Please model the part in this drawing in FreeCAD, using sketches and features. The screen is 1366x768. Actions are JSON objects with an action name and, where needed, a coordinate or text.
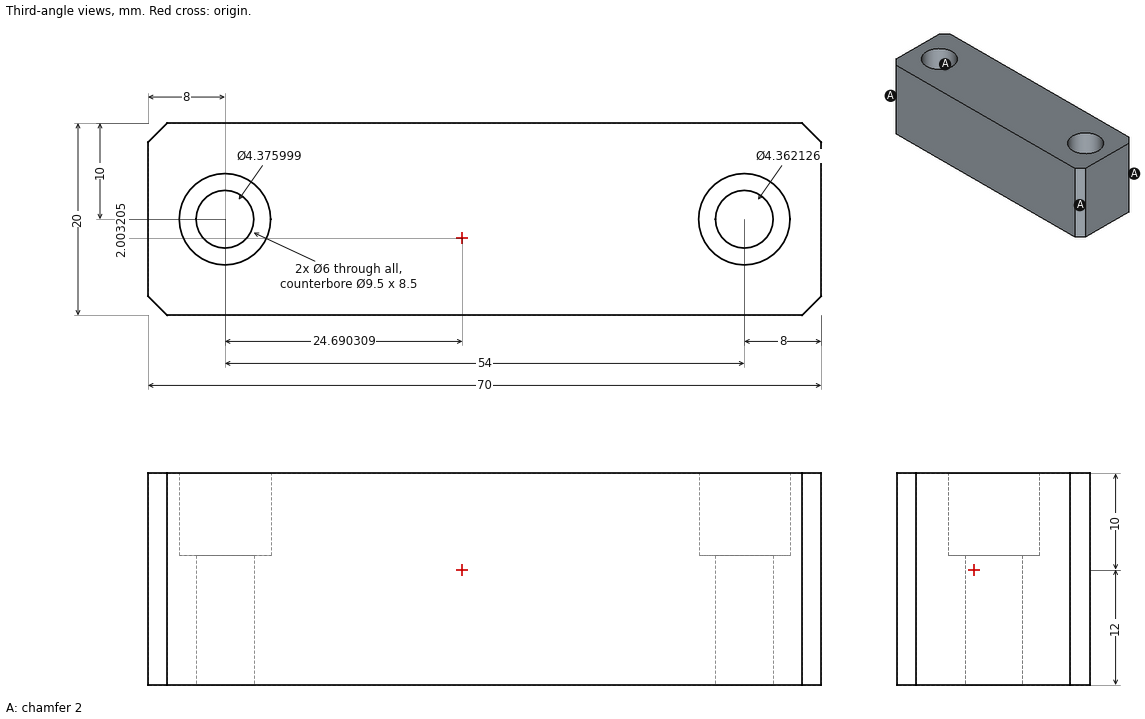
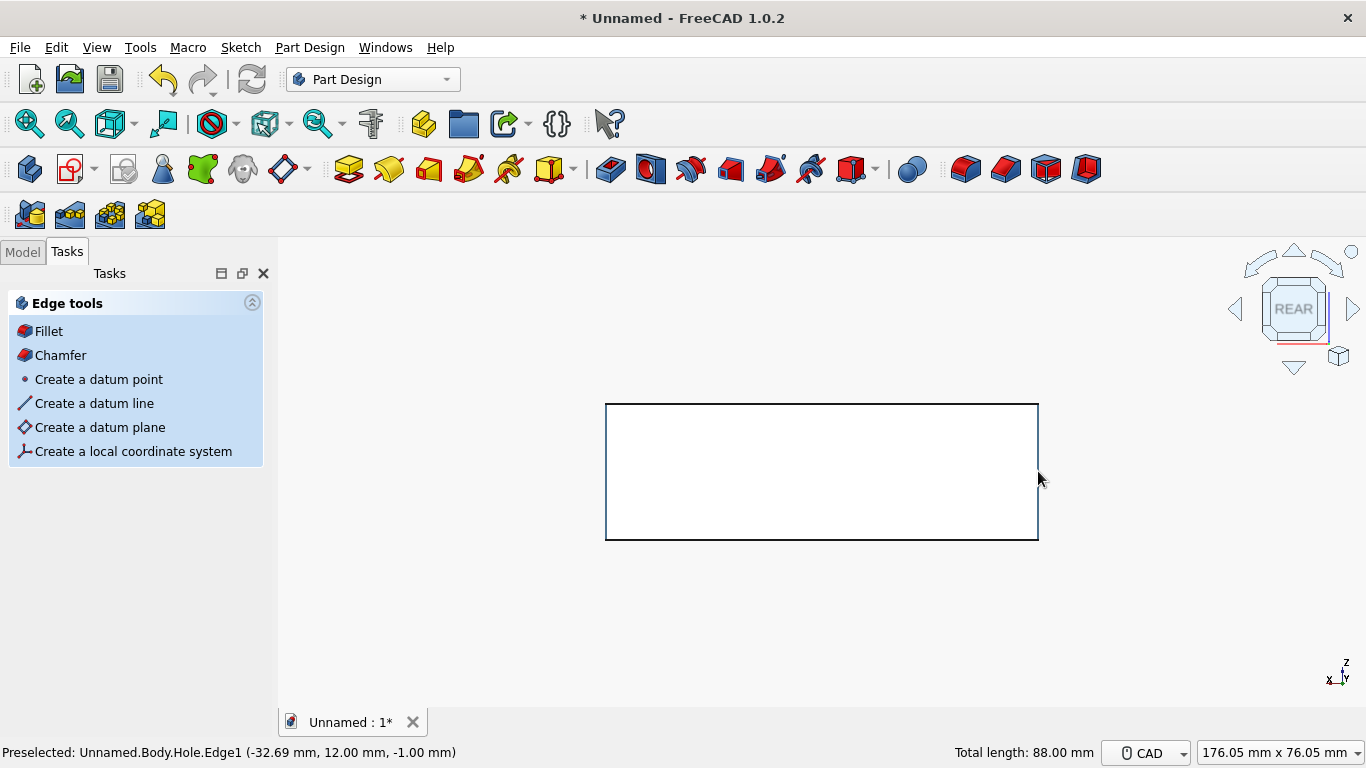
{"action": "left_click", "coordinate": [1006, 170]}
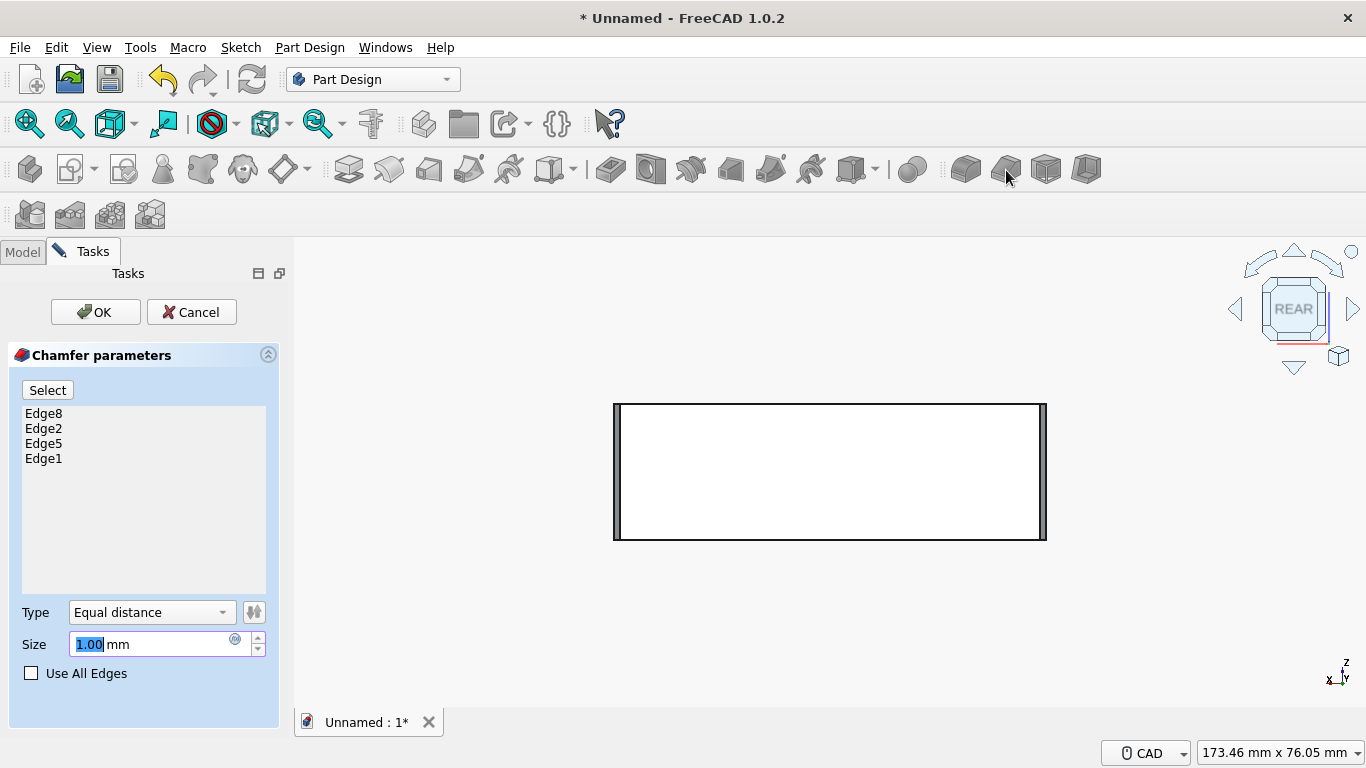
{"action": "type", "text": "2"}
{"action": "key", "text": "Tab"}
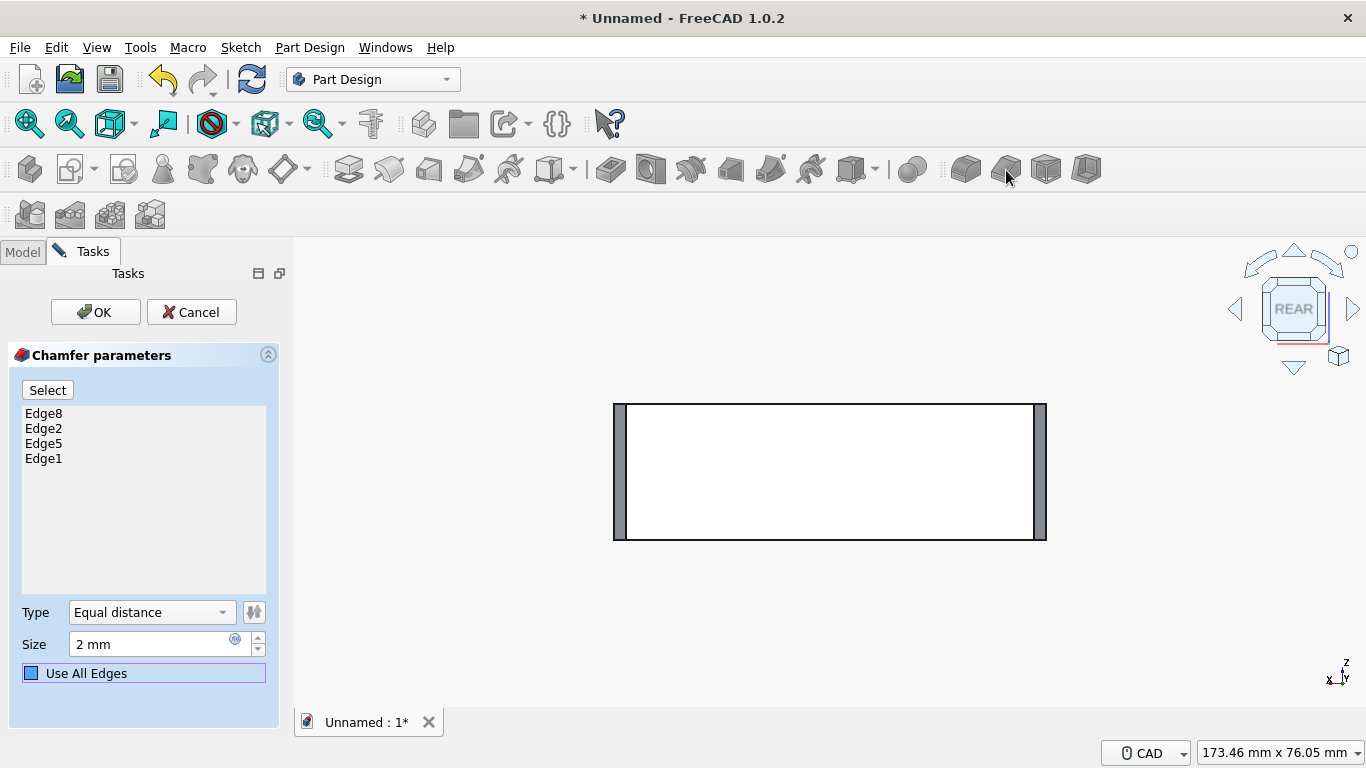
{"action": "left_click", "coordinate": [96, 312]}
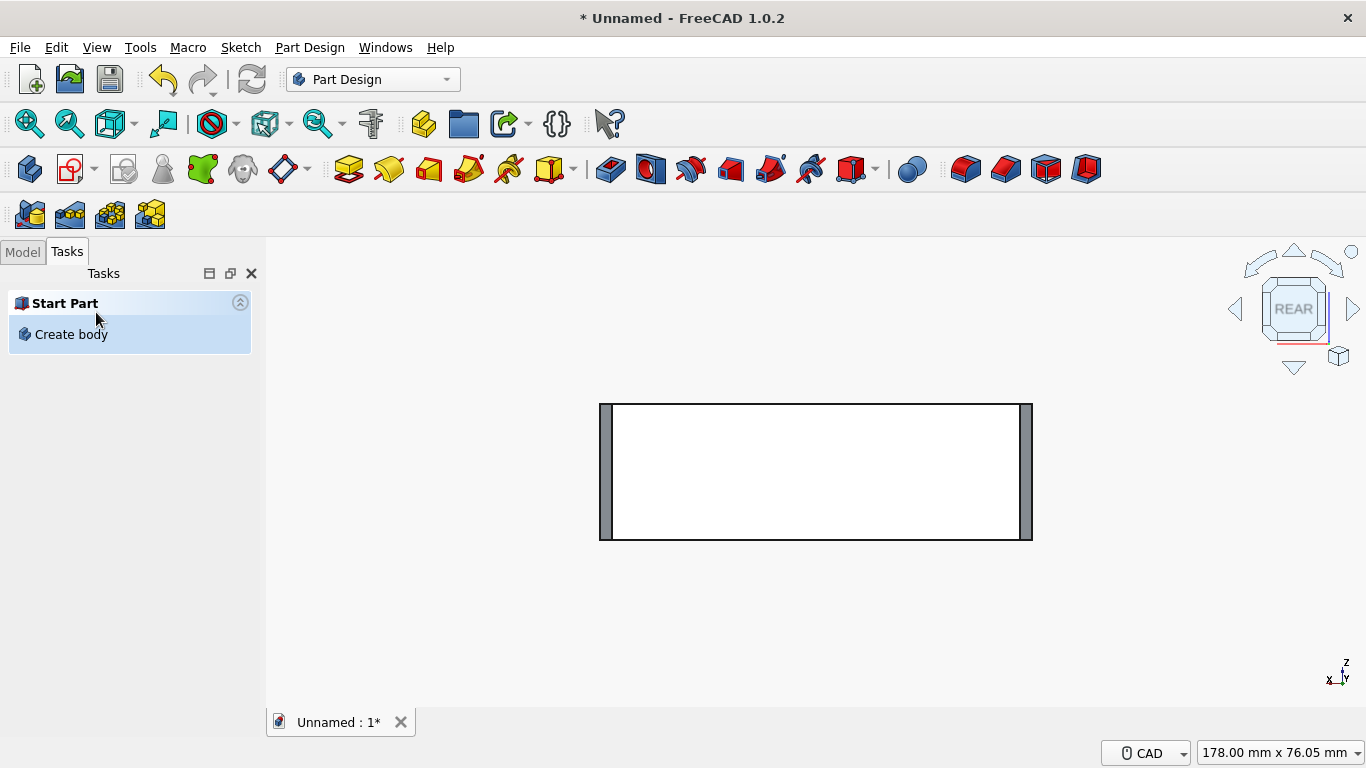
{"action": "key", "text": "0"}